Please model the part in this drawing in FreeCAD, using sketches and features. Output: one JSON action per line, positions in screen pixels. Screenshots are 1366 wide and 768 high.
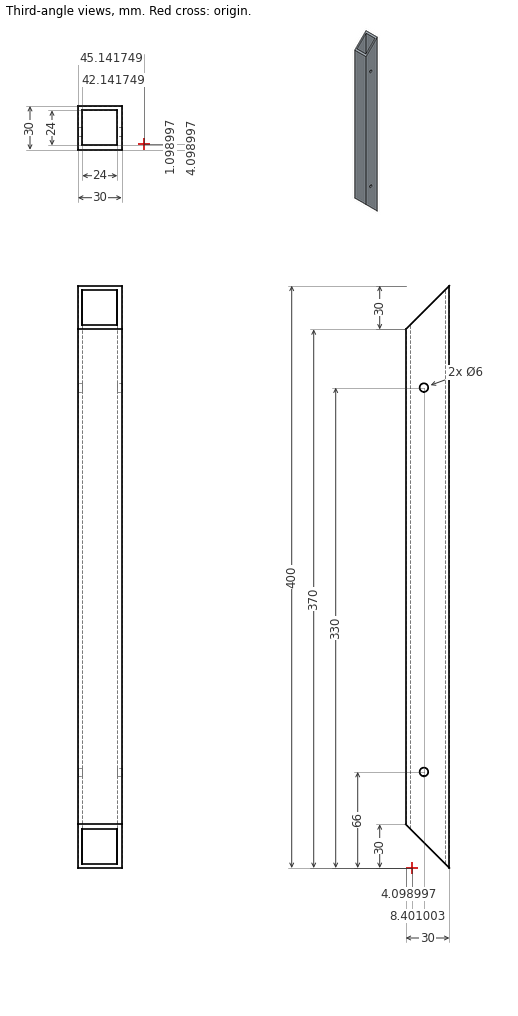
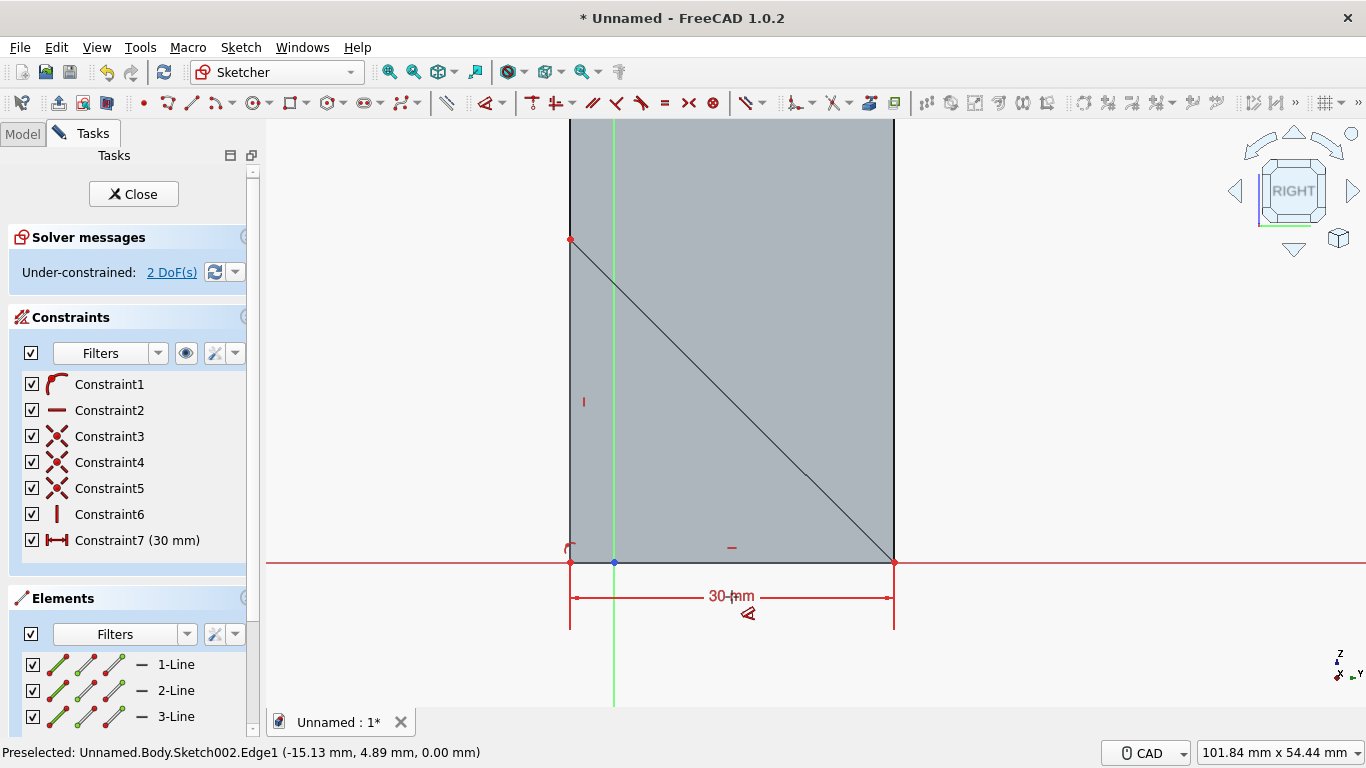
{"action": "left_click", "coordinate": [570, 337]}
{"action": "left_click", "coordinate": [536, 401]}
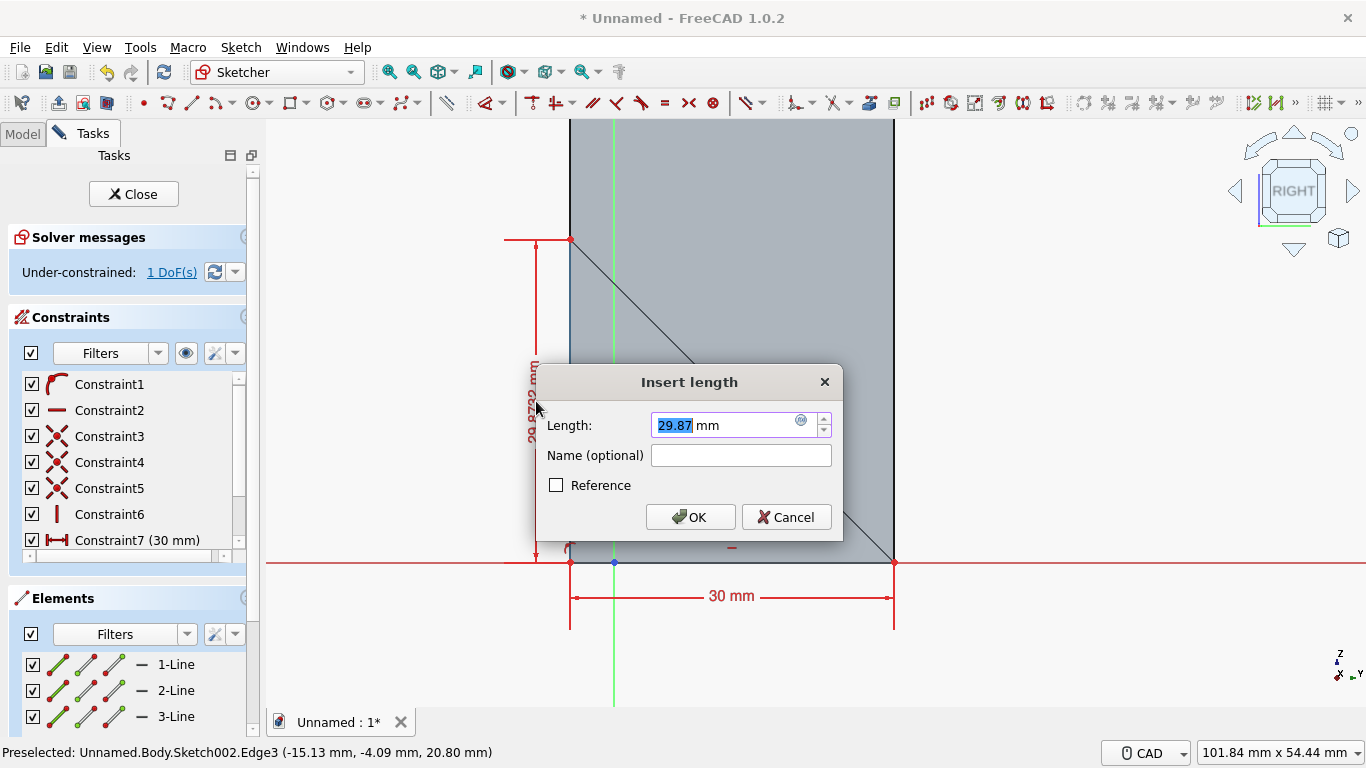
{"action": "type", "text": "30"}
{"action": "key", "text": "Return"}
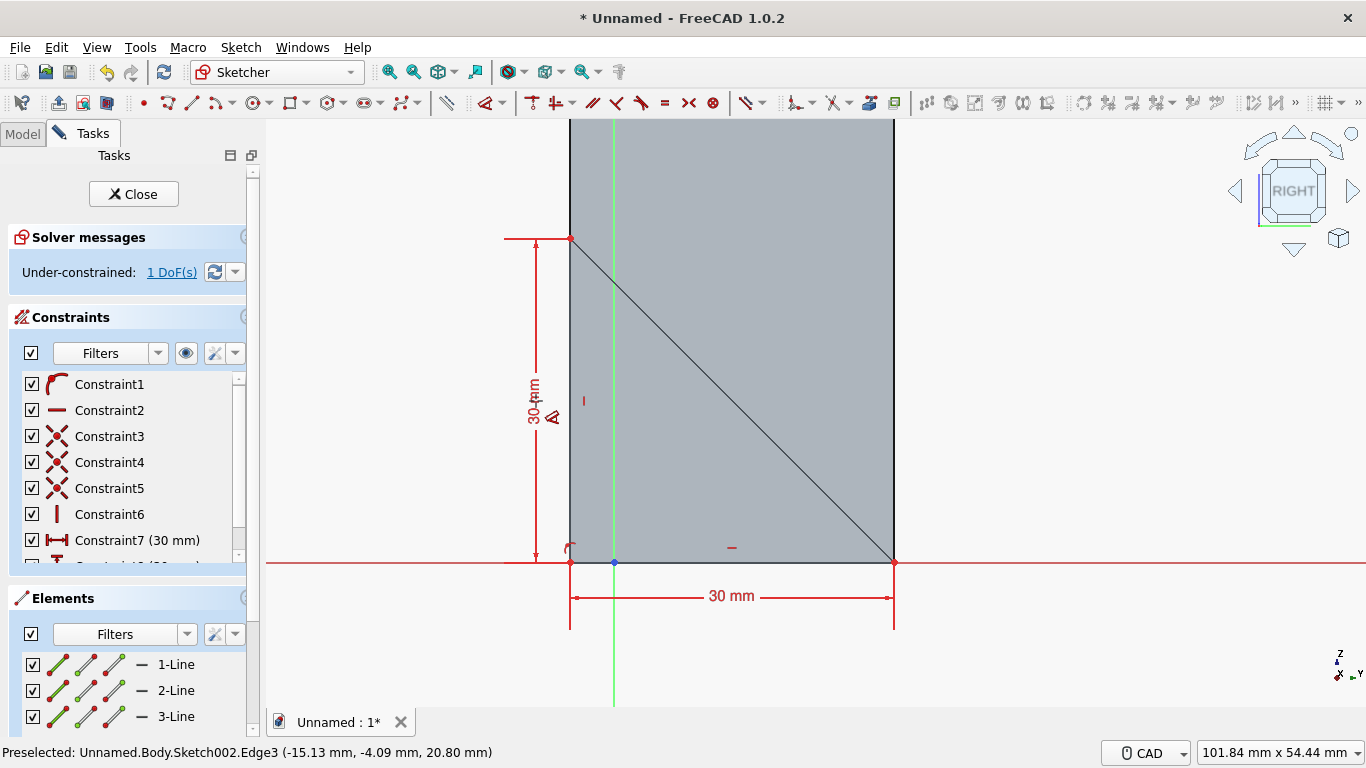
{"action": "left_click", "coordinate": [570, 563]}
{"action": "left_click", "coordinate": [592, 597]}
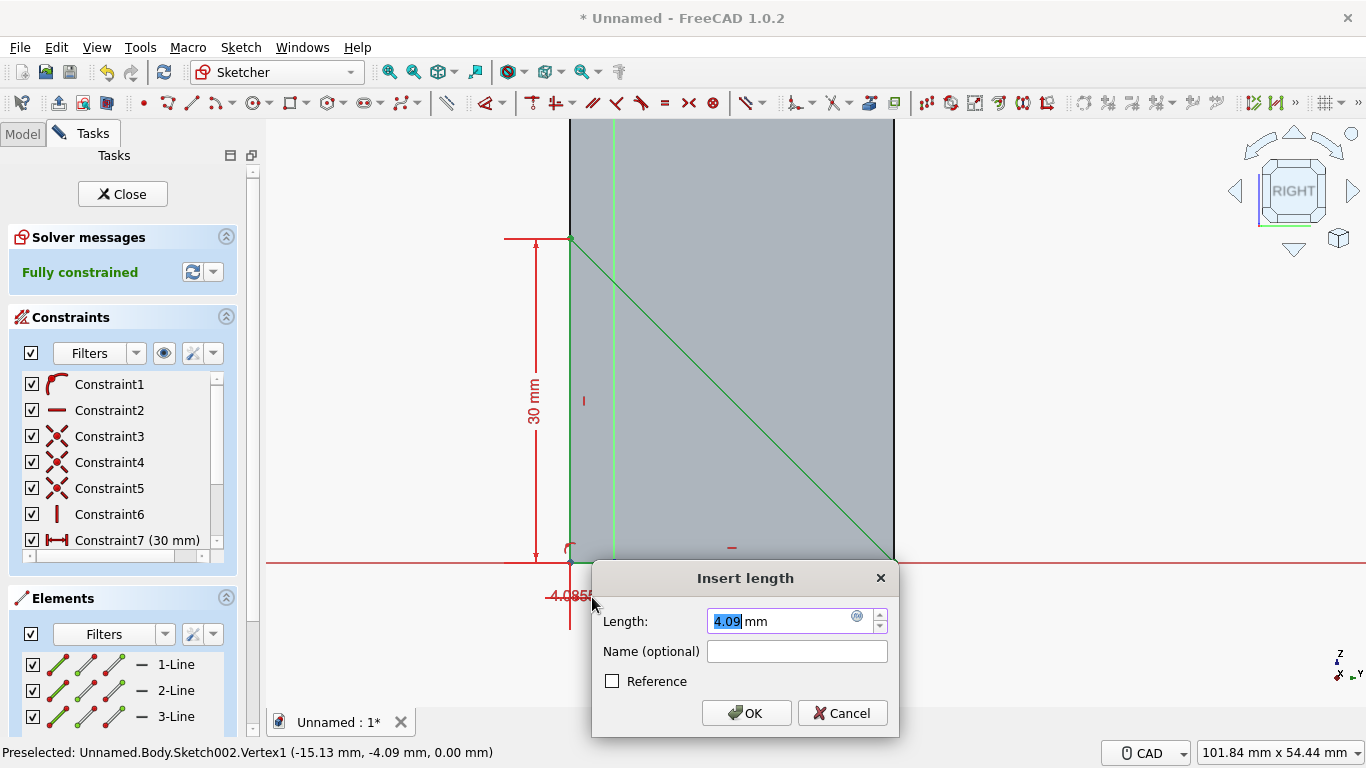
{"action": "type", "text": "4.098997"}
{"action": "key", "text": "Return"}
{"action": "key", "text": "Escape"}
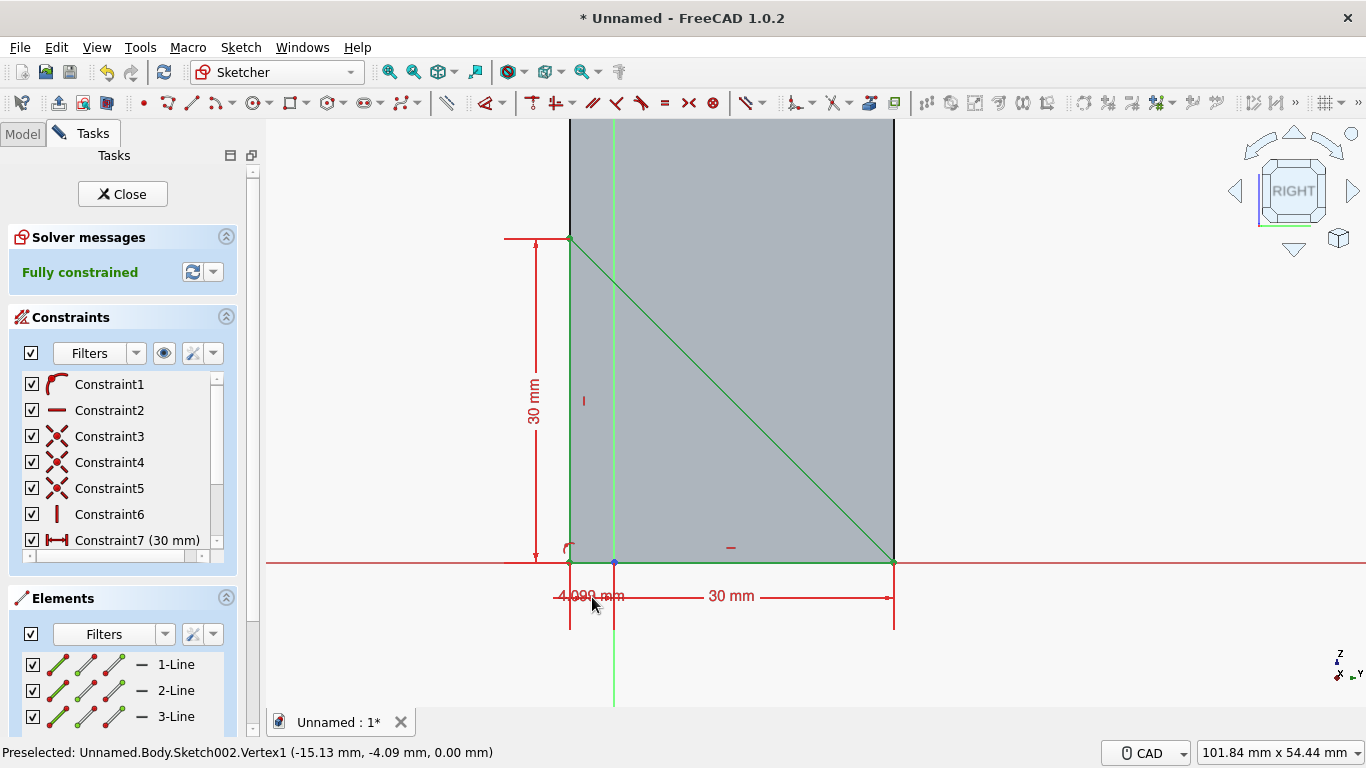
{"action": "left_click", "coordinate": [123, 194]}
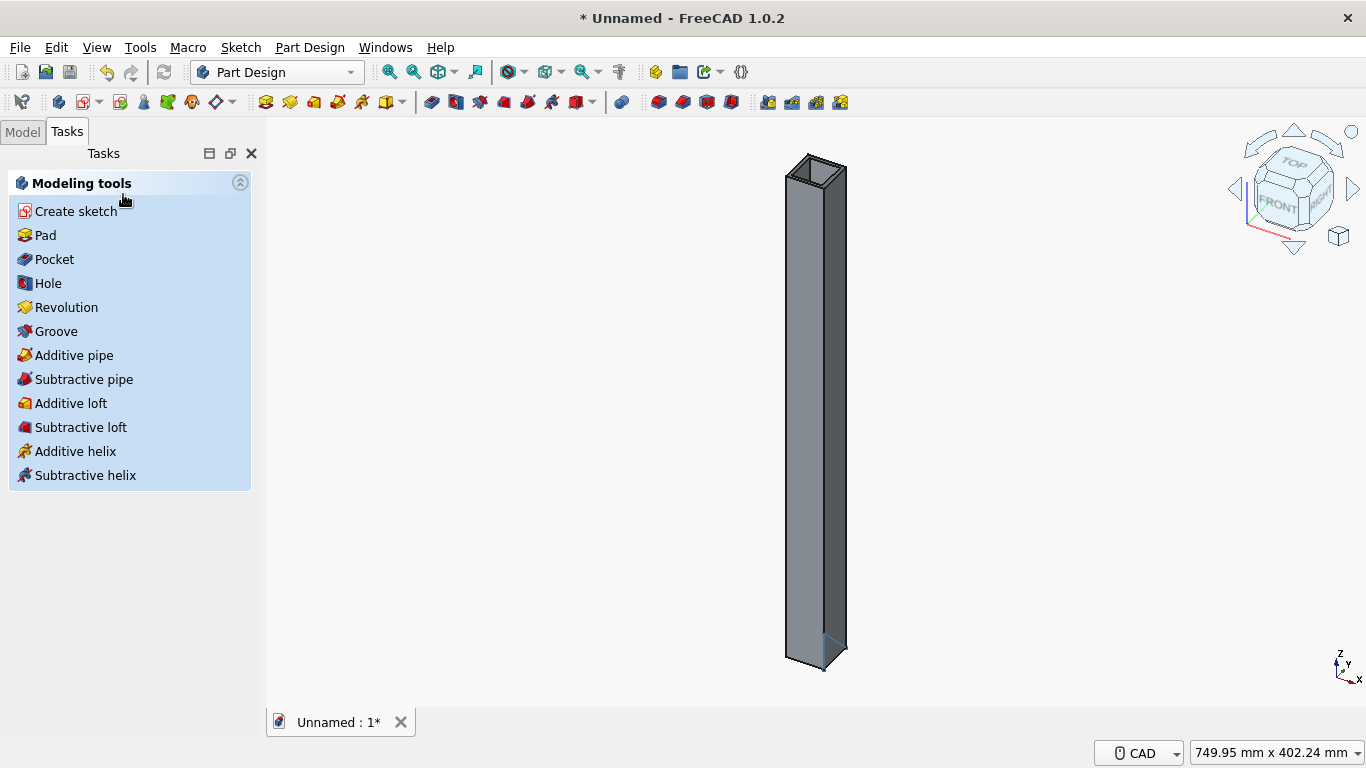
{"action": "left_click", "coordinate": [432, 102]}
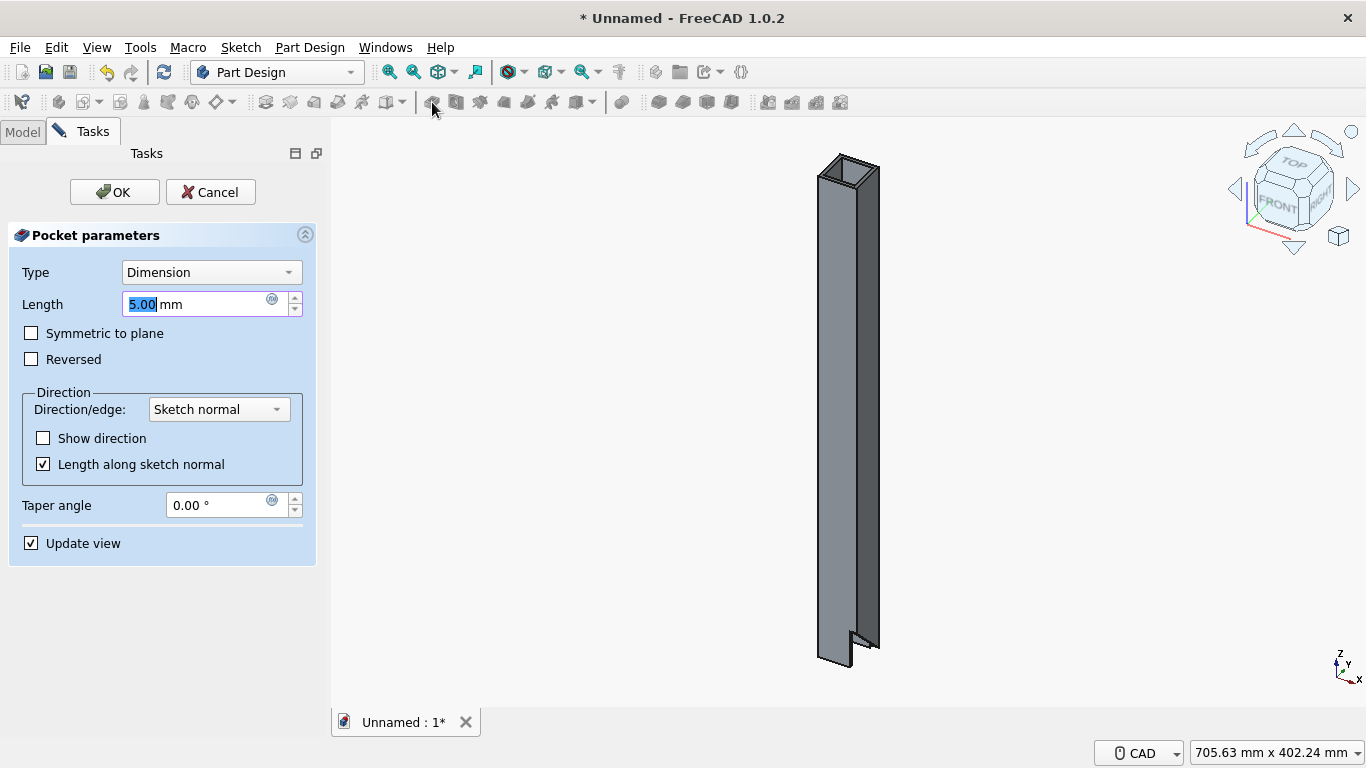
{"action": "left_click", "coordinate": [212, 272]}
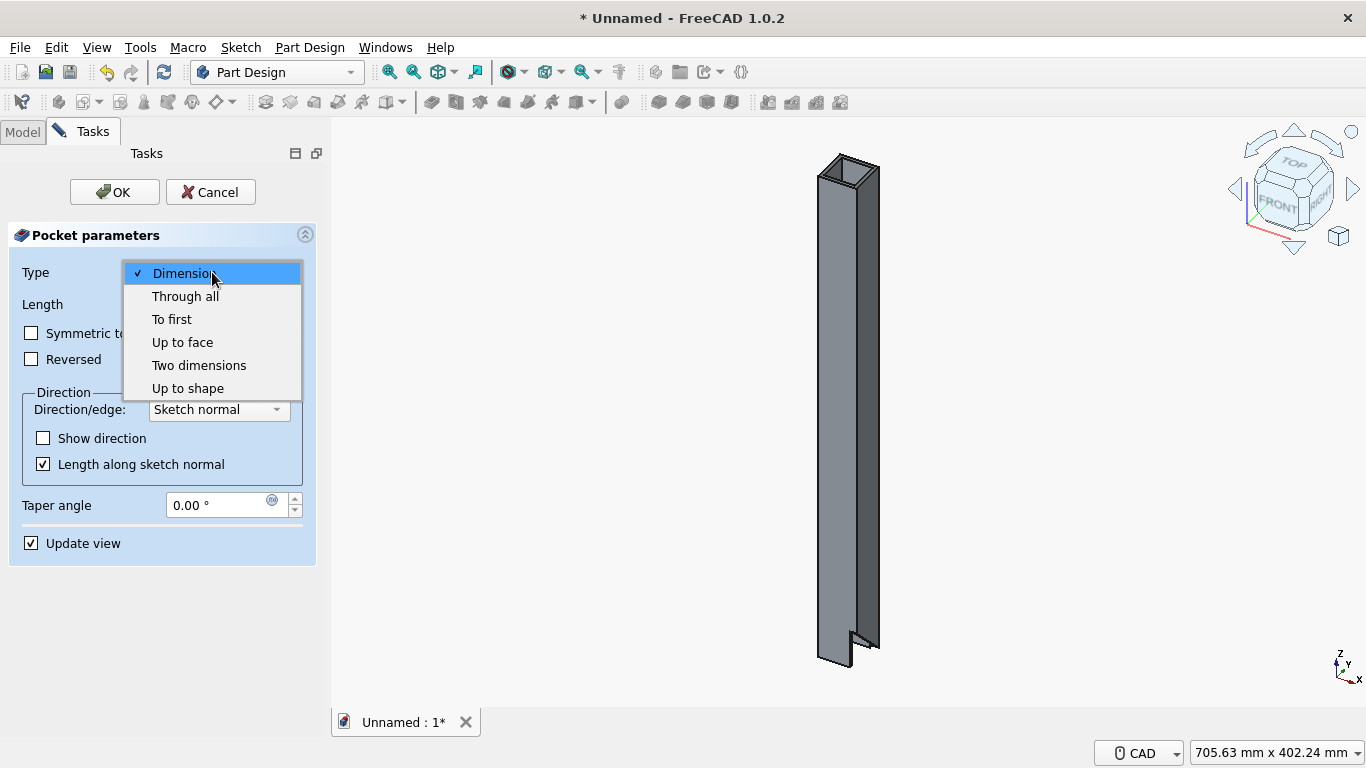
{"action": "left_click", "coordinate": [212, 296]}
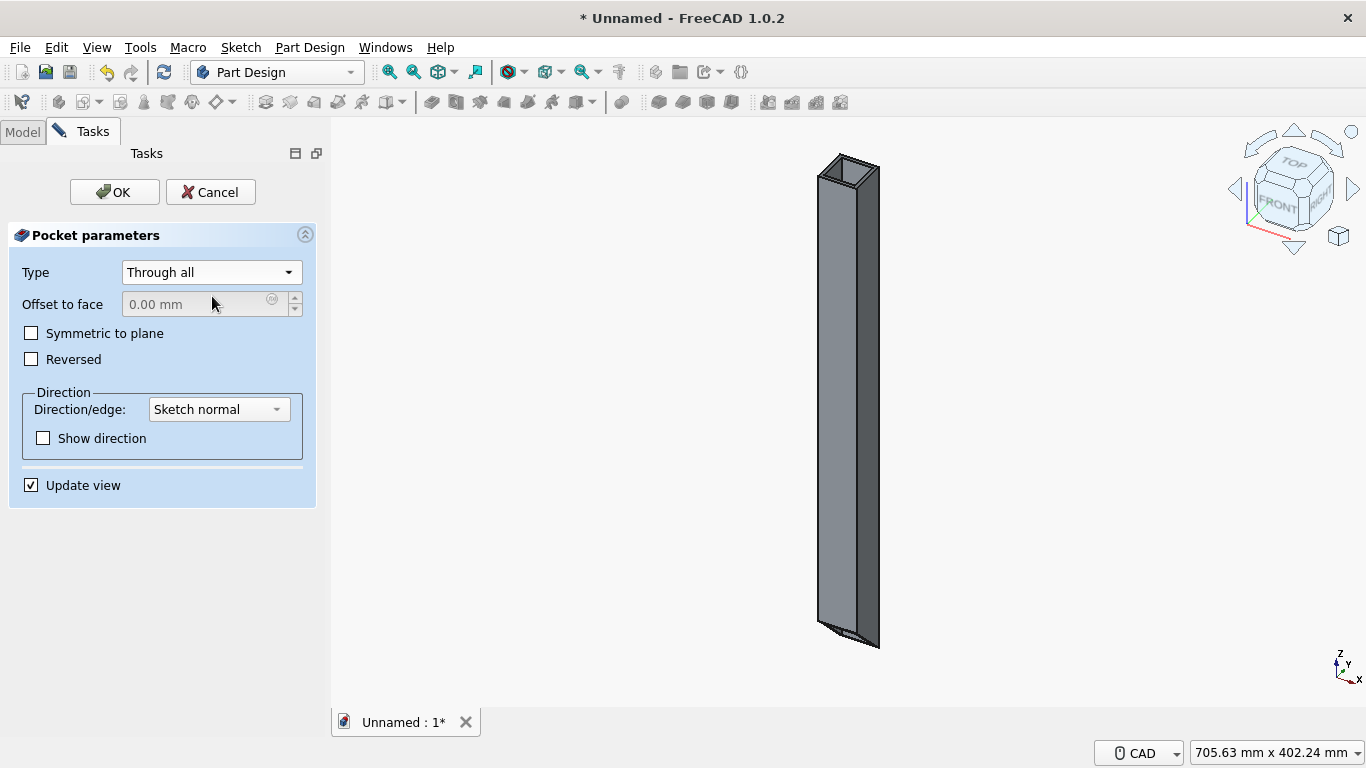
{"action": "left_click", "coordinate": [115, 192]}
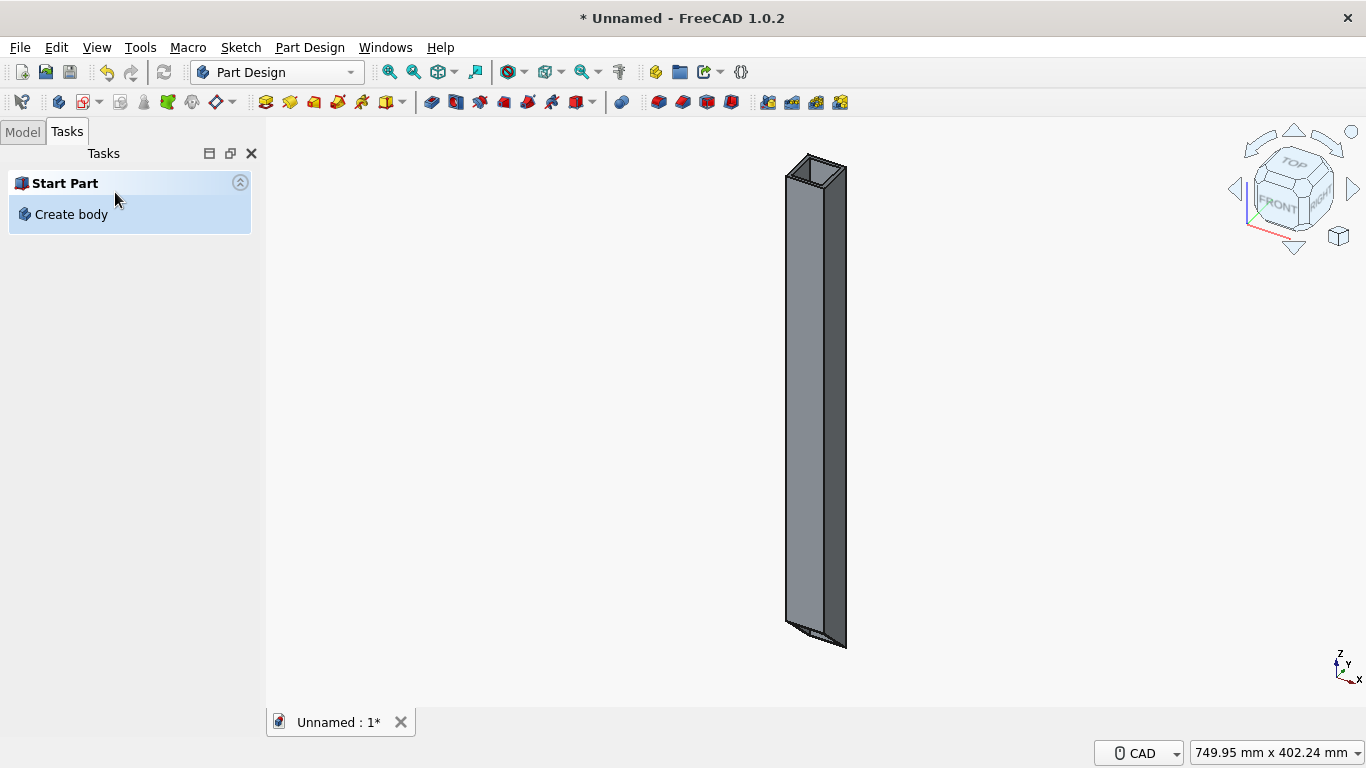
{"action": "left_click", "coordinate": [835, 211]}